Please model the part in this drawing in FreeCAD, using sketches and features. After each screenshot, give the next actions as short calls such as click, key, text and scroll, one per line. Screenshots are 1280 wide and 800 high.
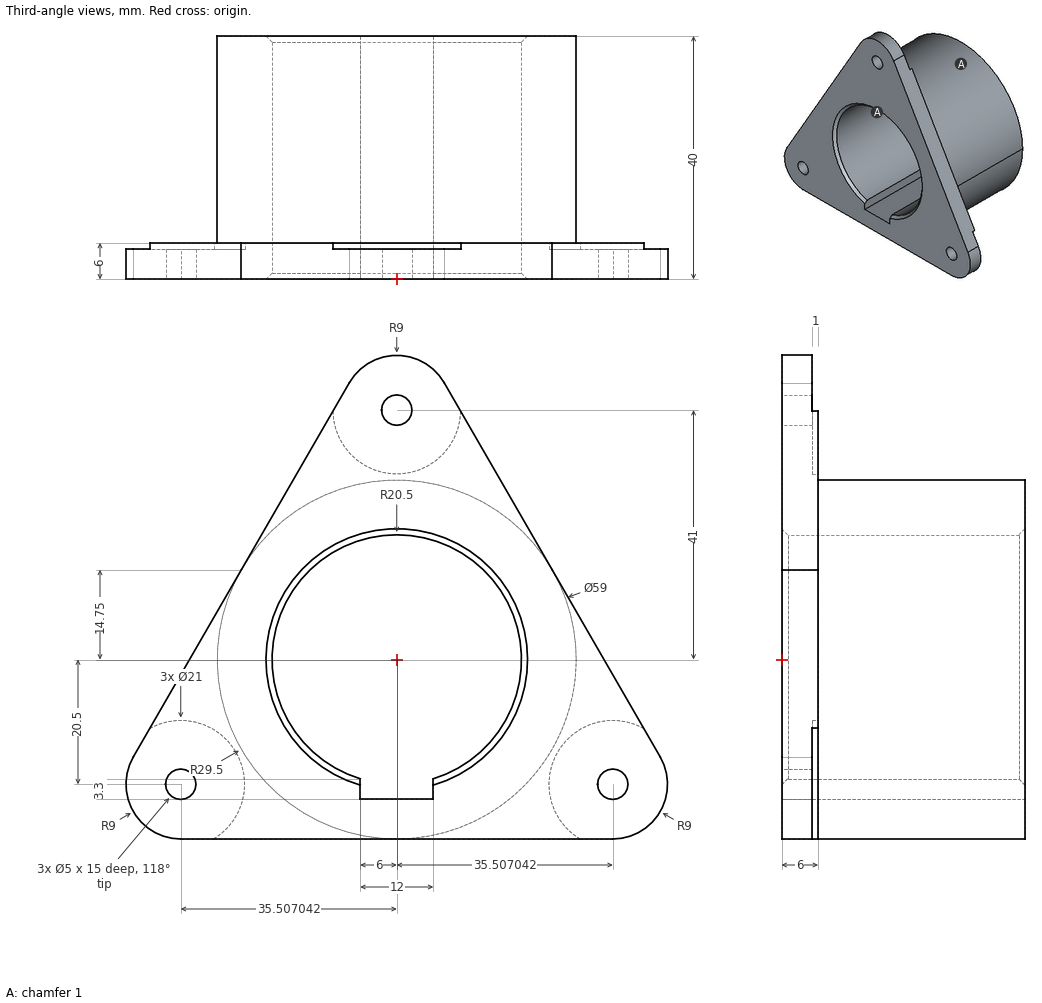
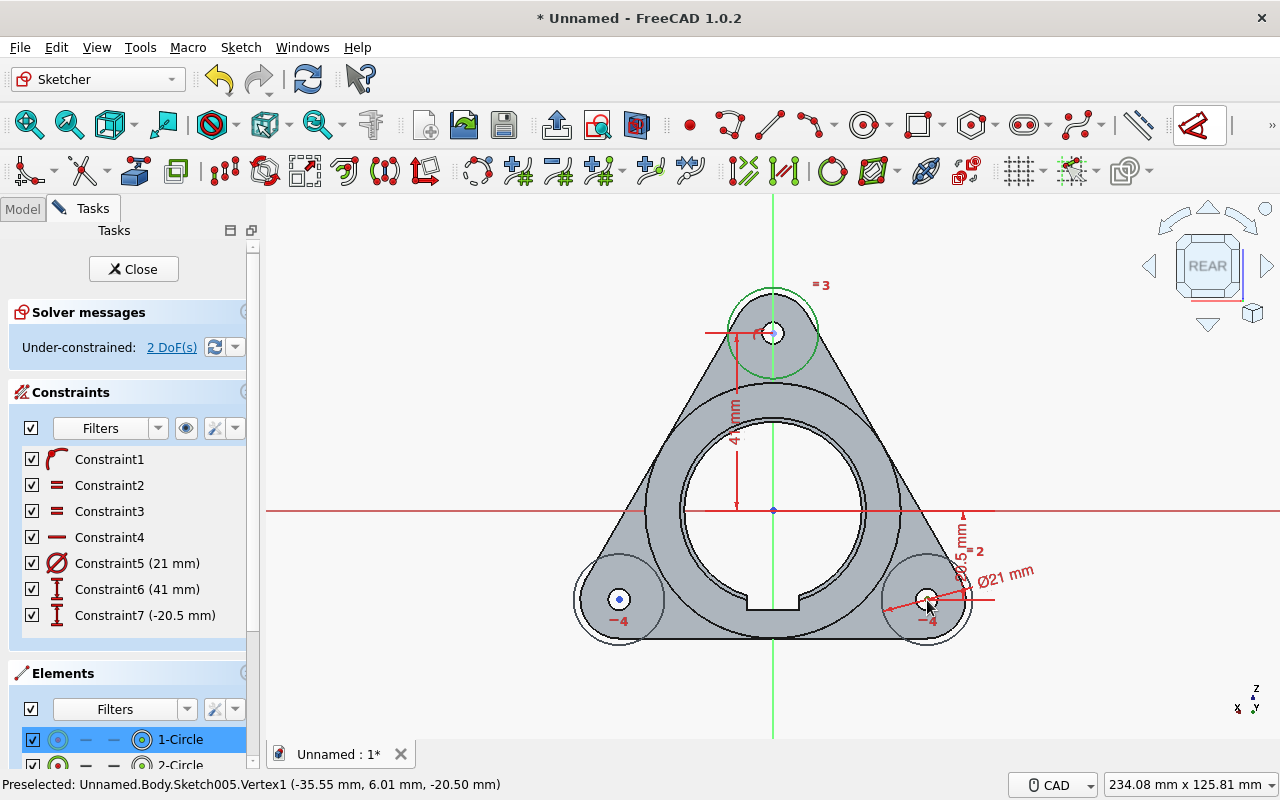
click(1220, 126)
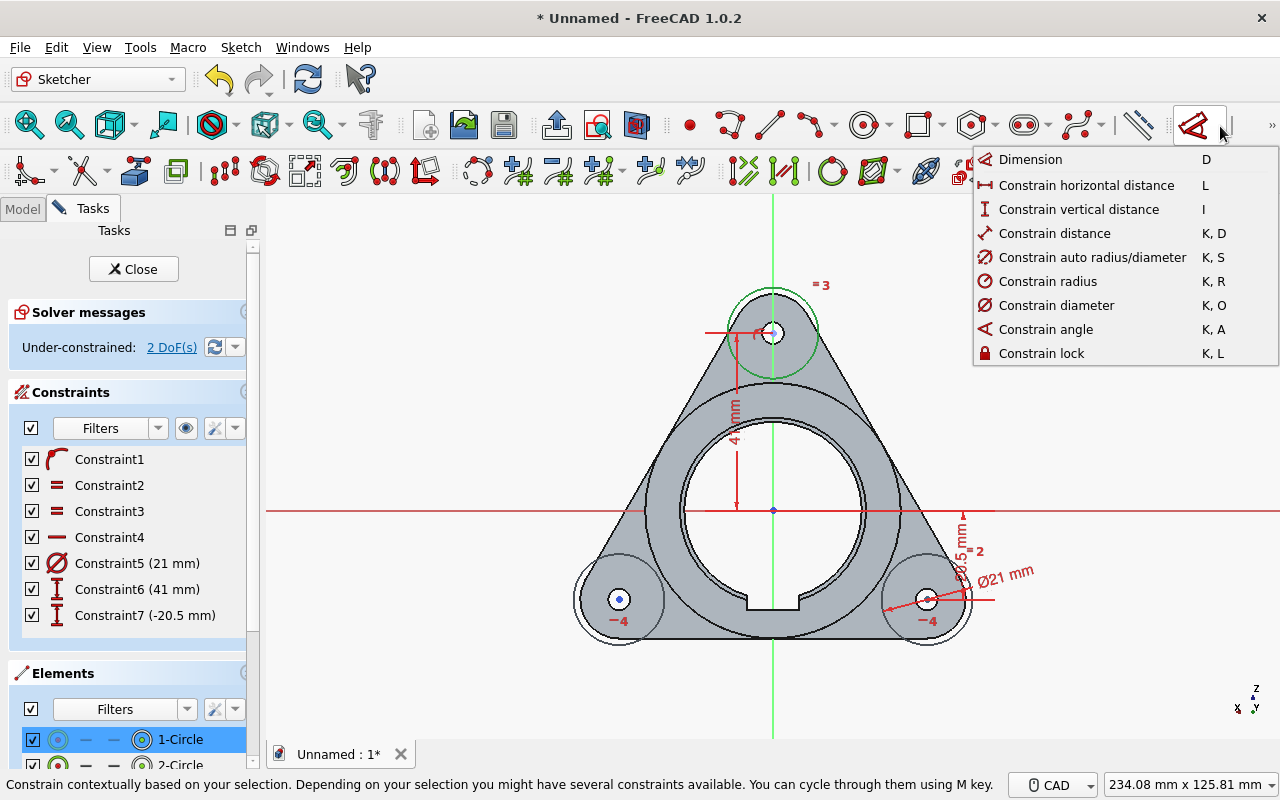
click(1126, 185)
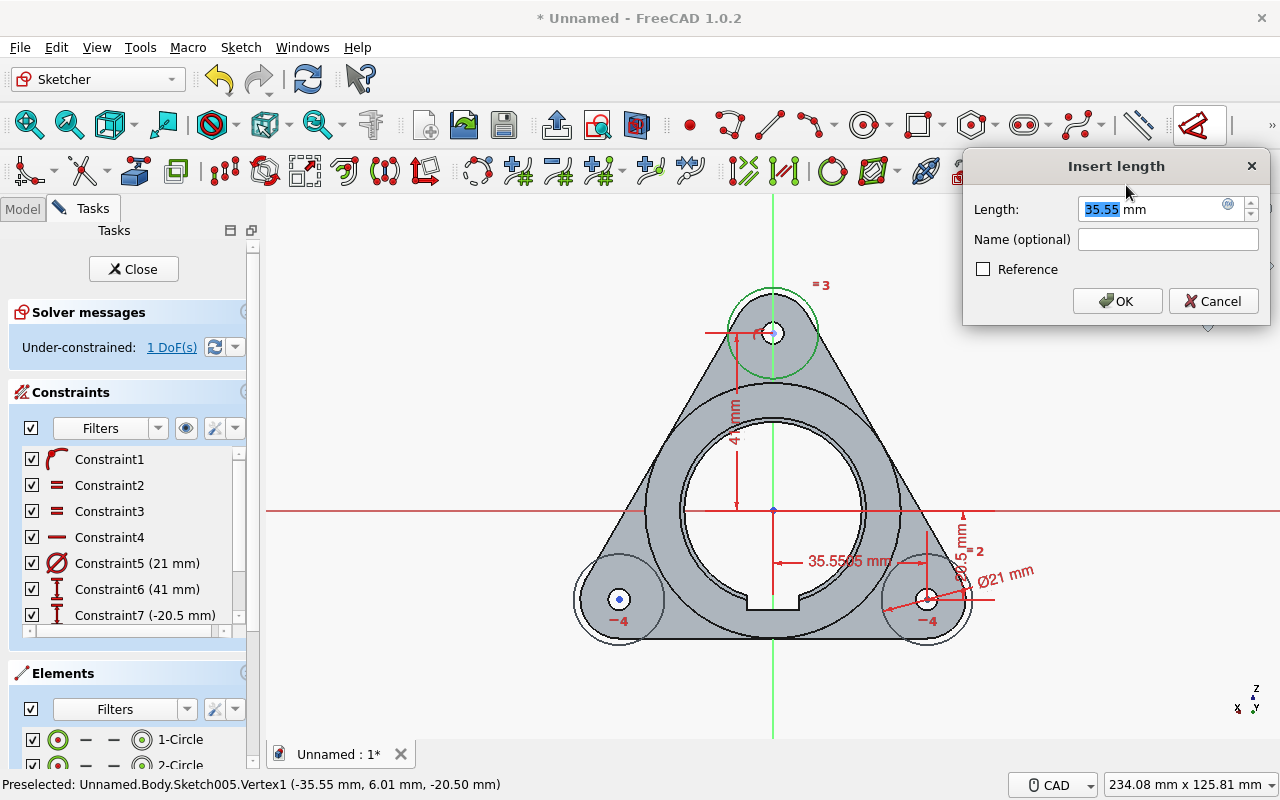
text(35.507042)
key(Return)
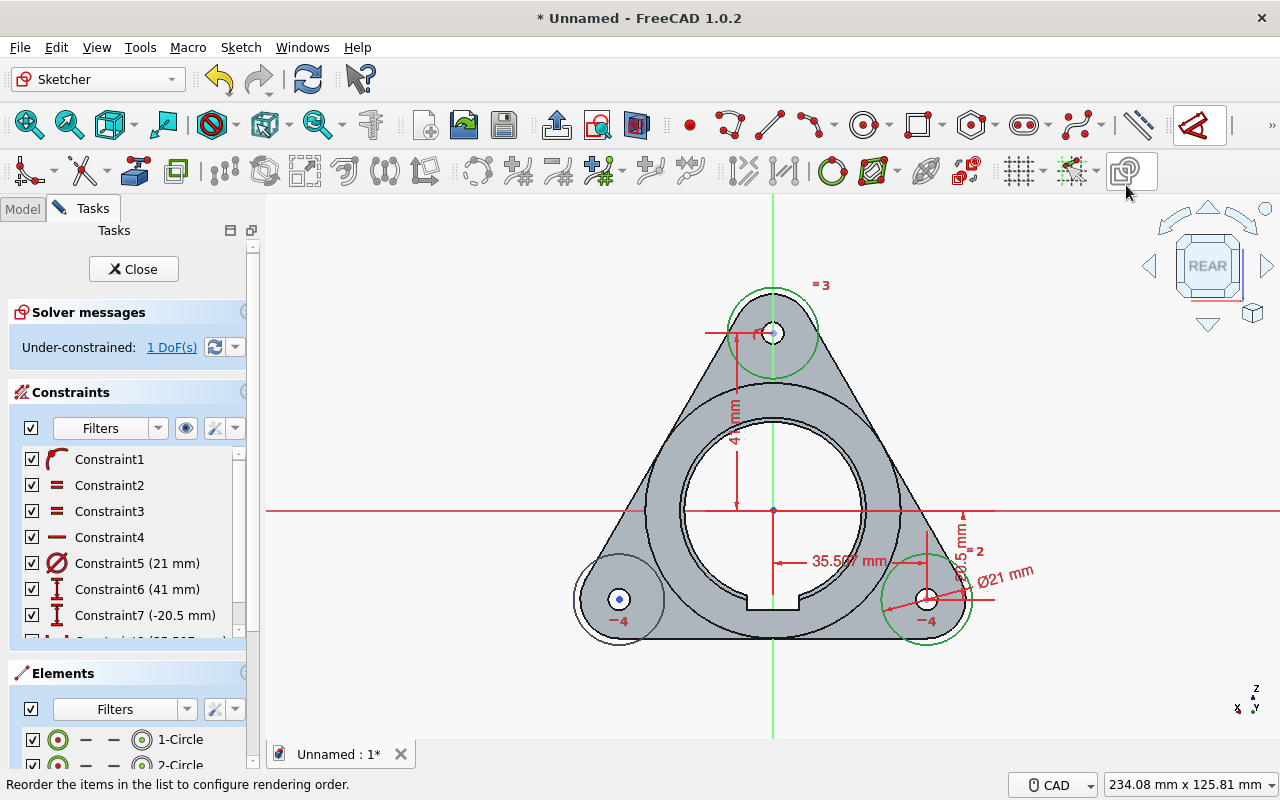
click(619, 600)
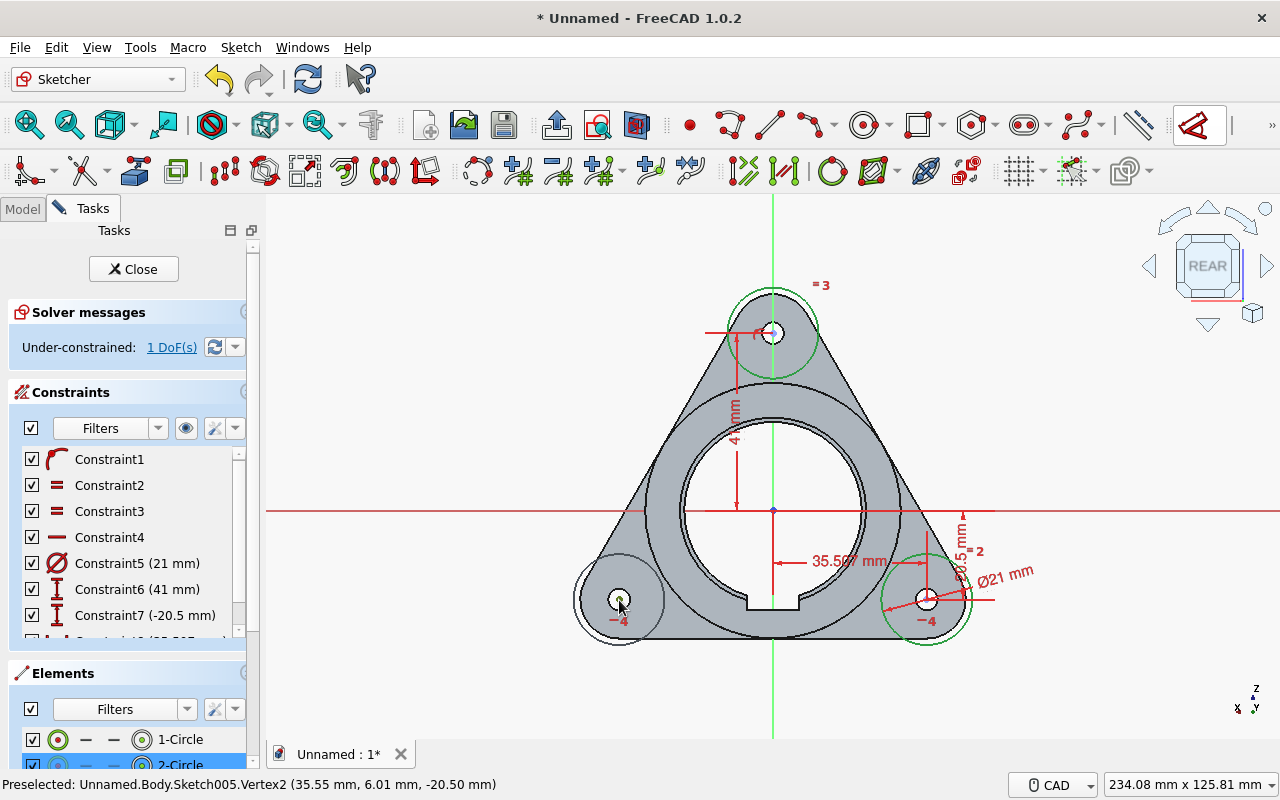
key(l)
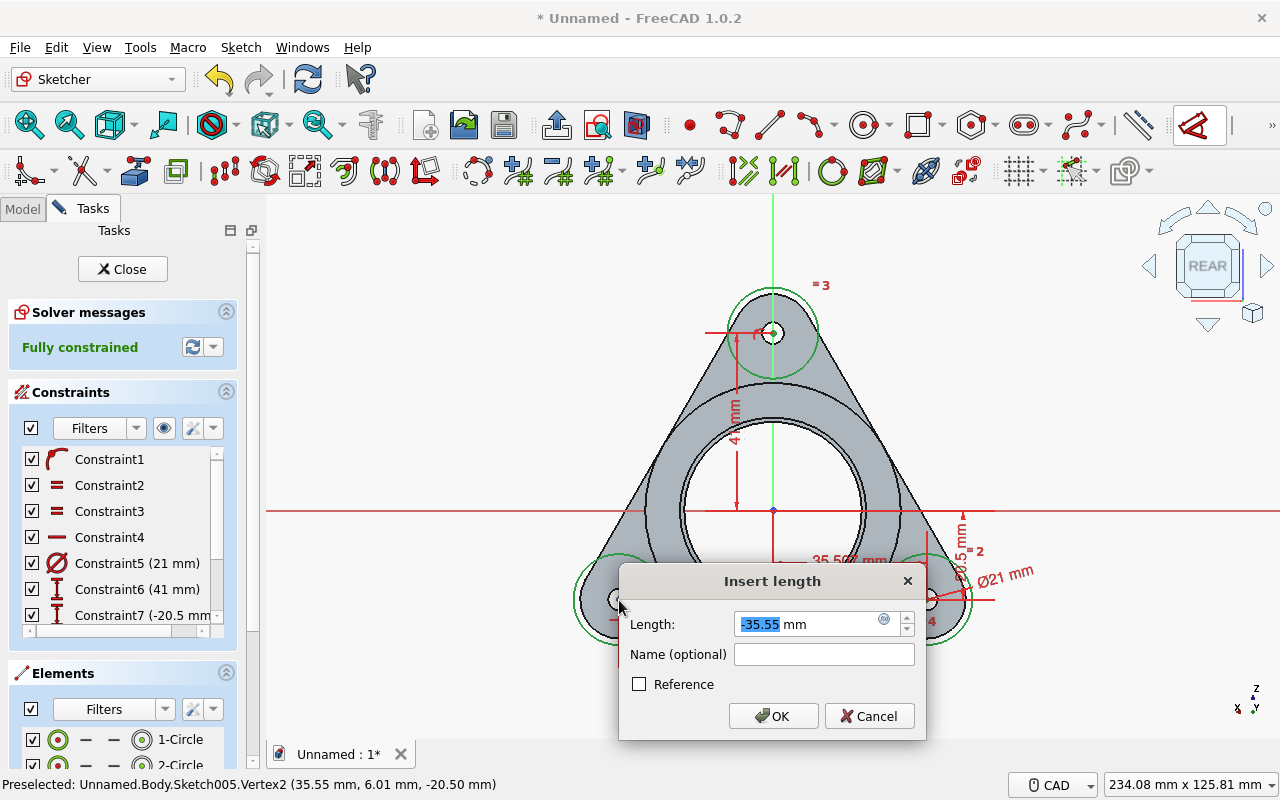
text(-35.507042)
key(Return)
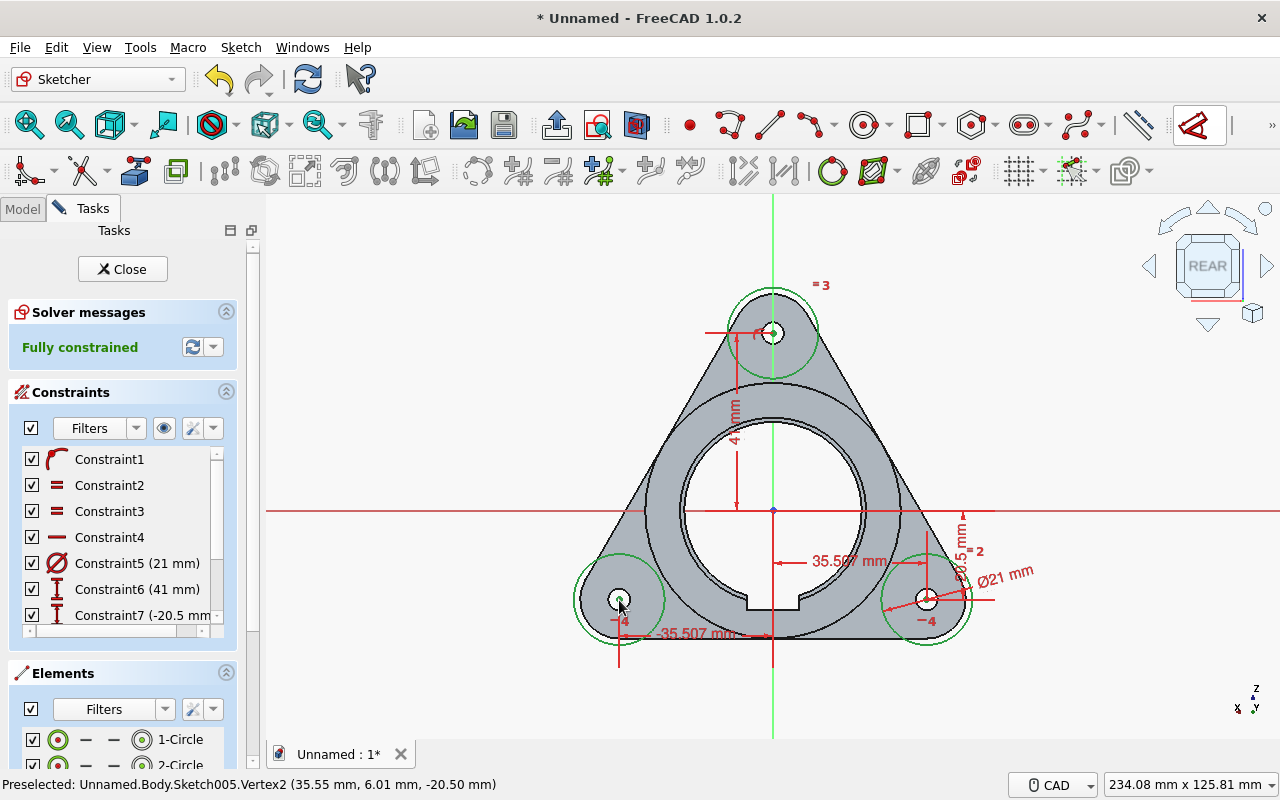
click(123, 269)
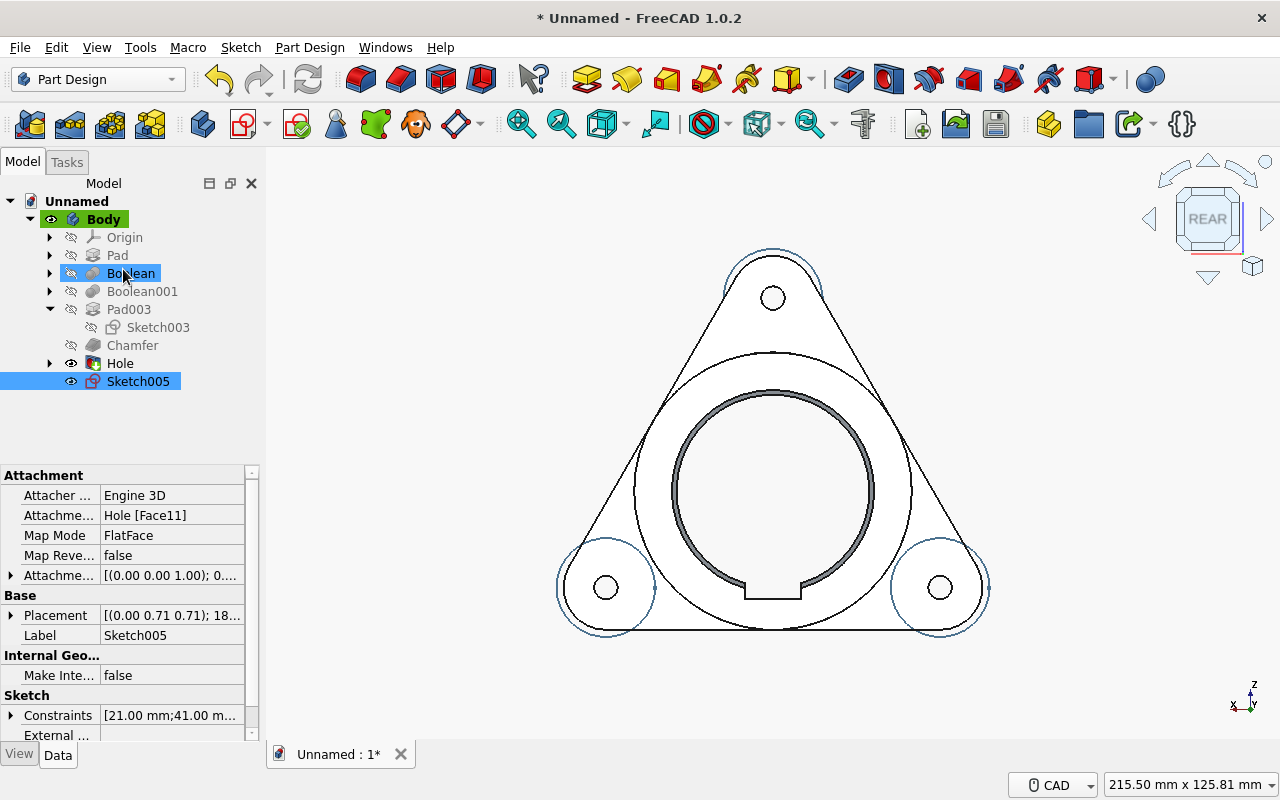
click(850, 80)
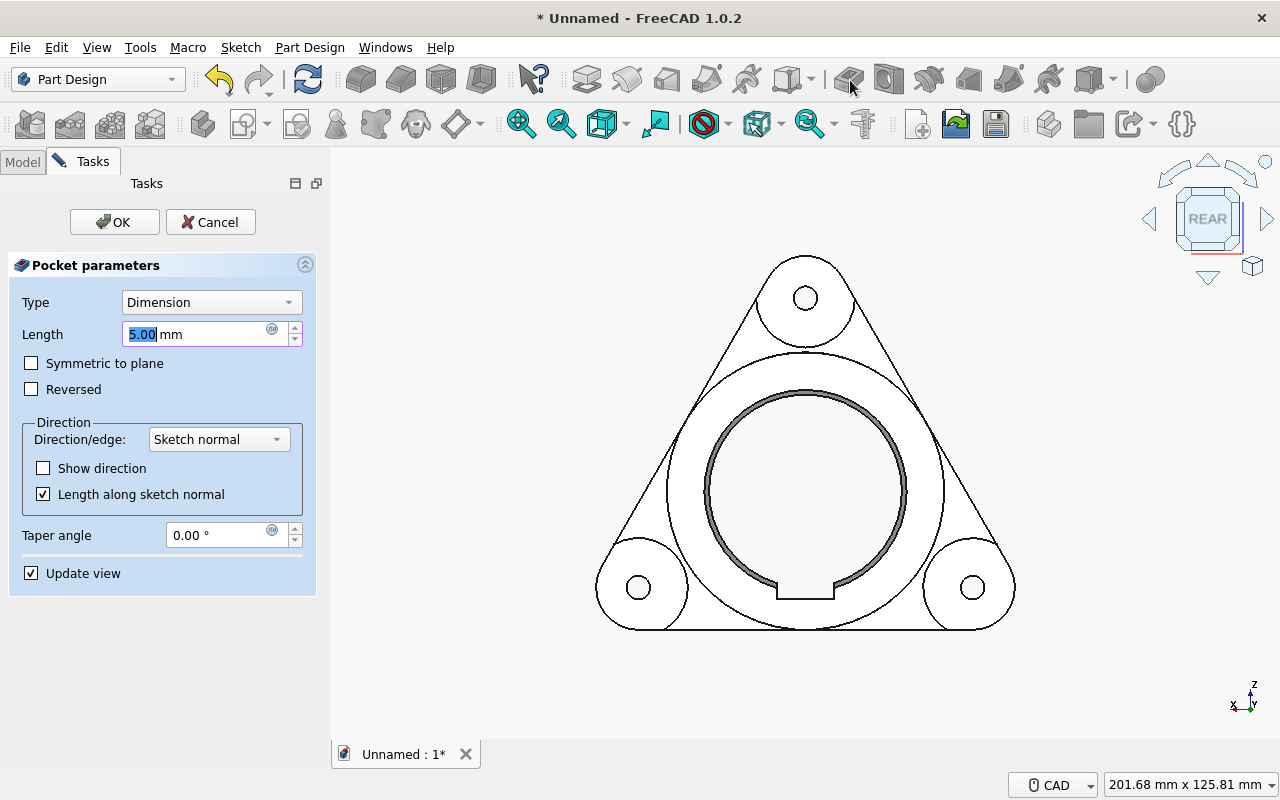
text(1)
key(Tab)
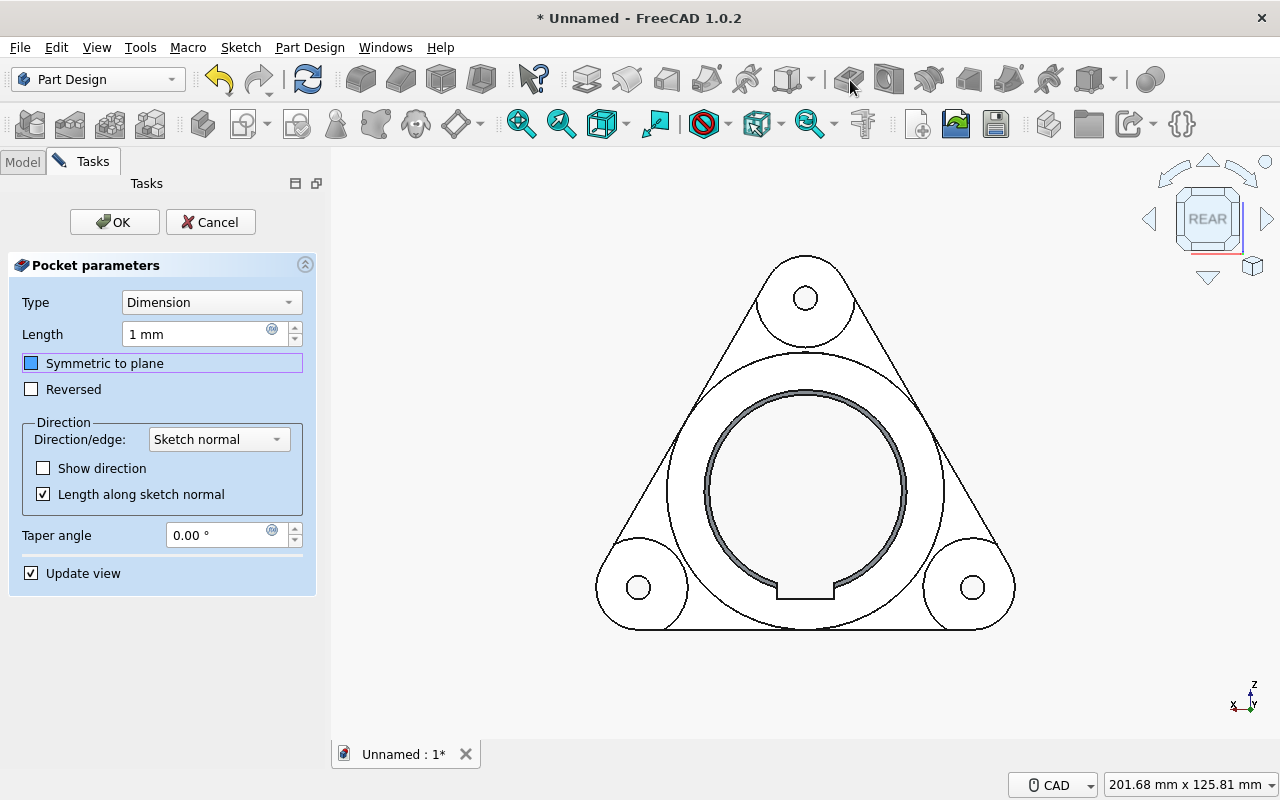
click(115, 222)